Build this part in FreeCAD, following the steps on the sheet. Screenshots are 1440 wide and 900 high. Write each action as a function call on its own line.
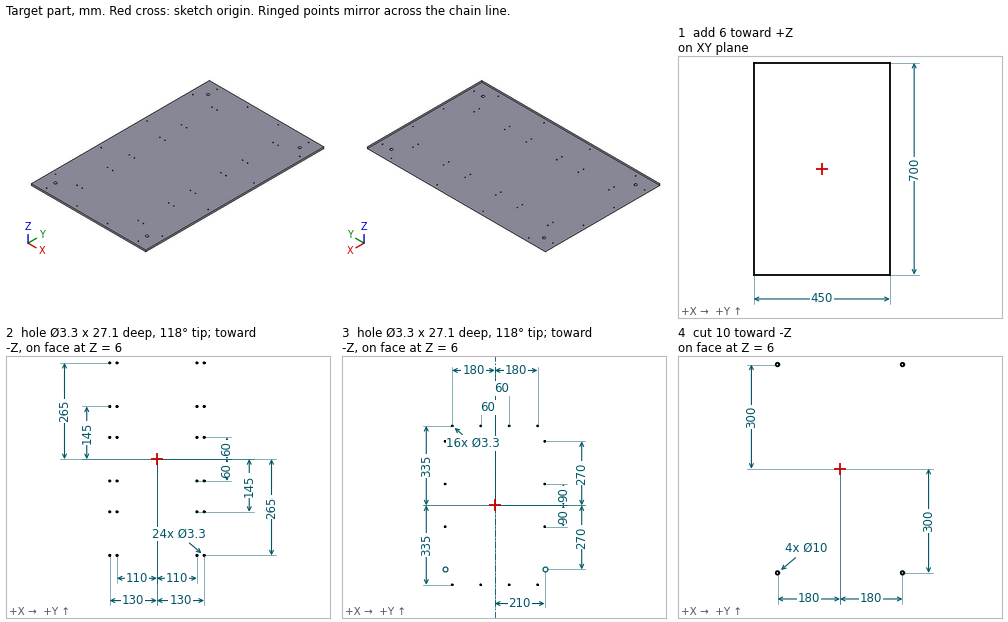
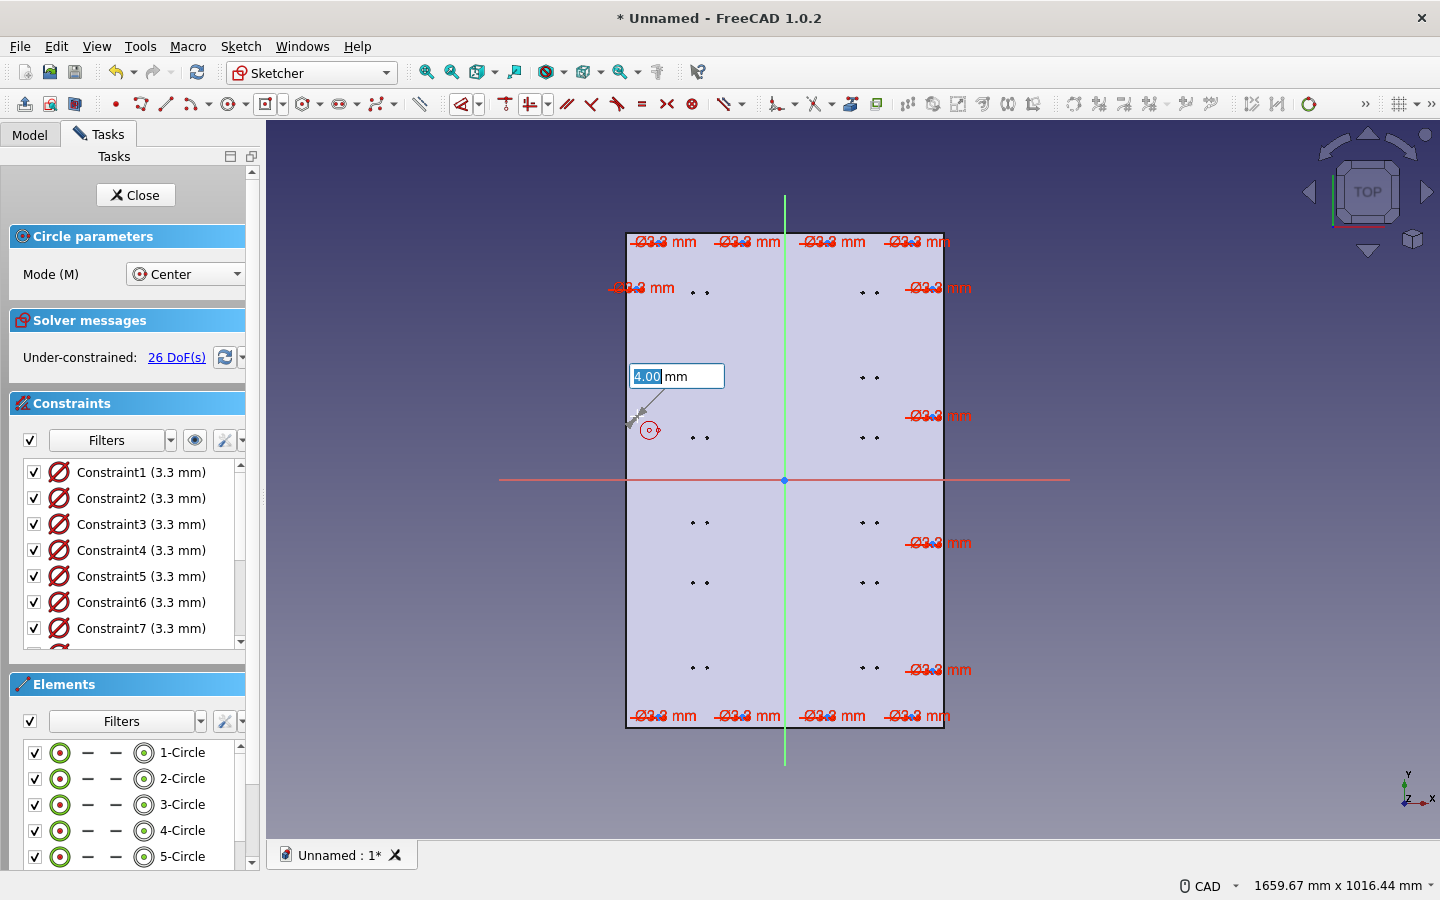
text(3.3)
key(Return)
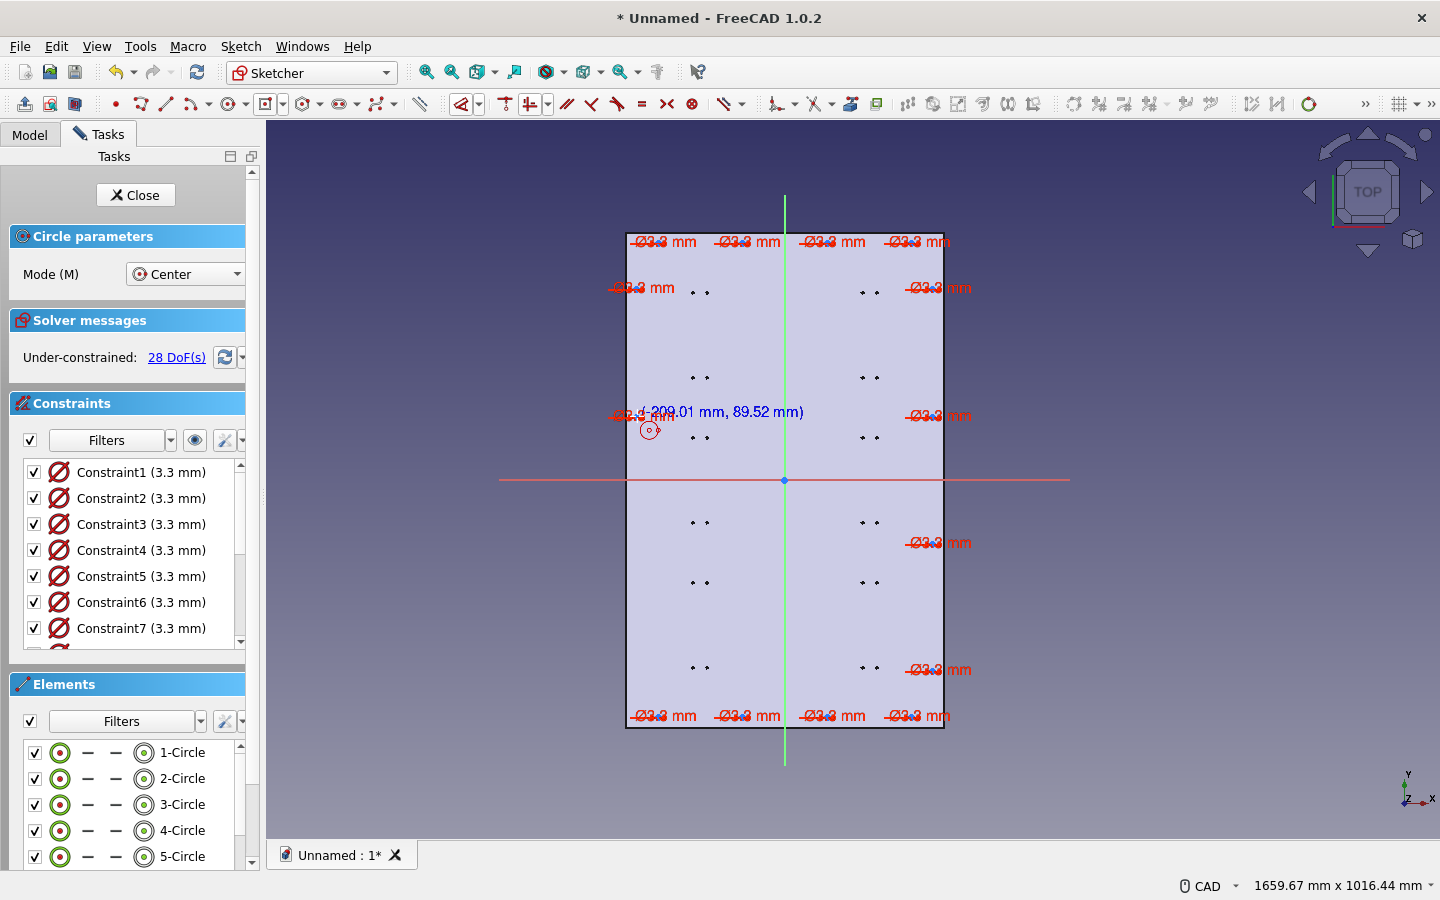
scroll(636, 544, up, 15)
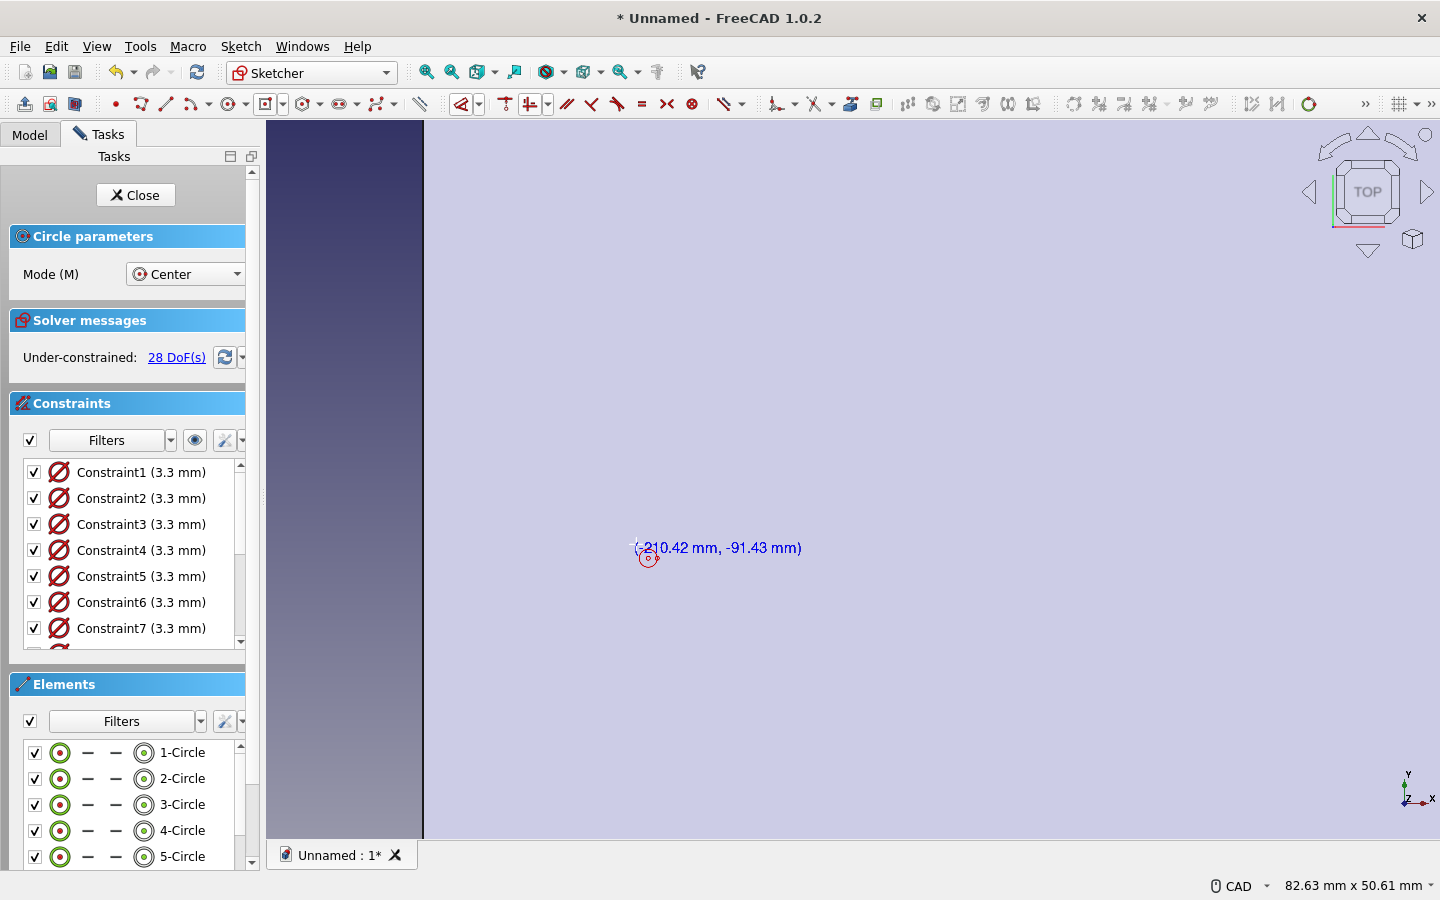
scroll(636, 544, down, 15)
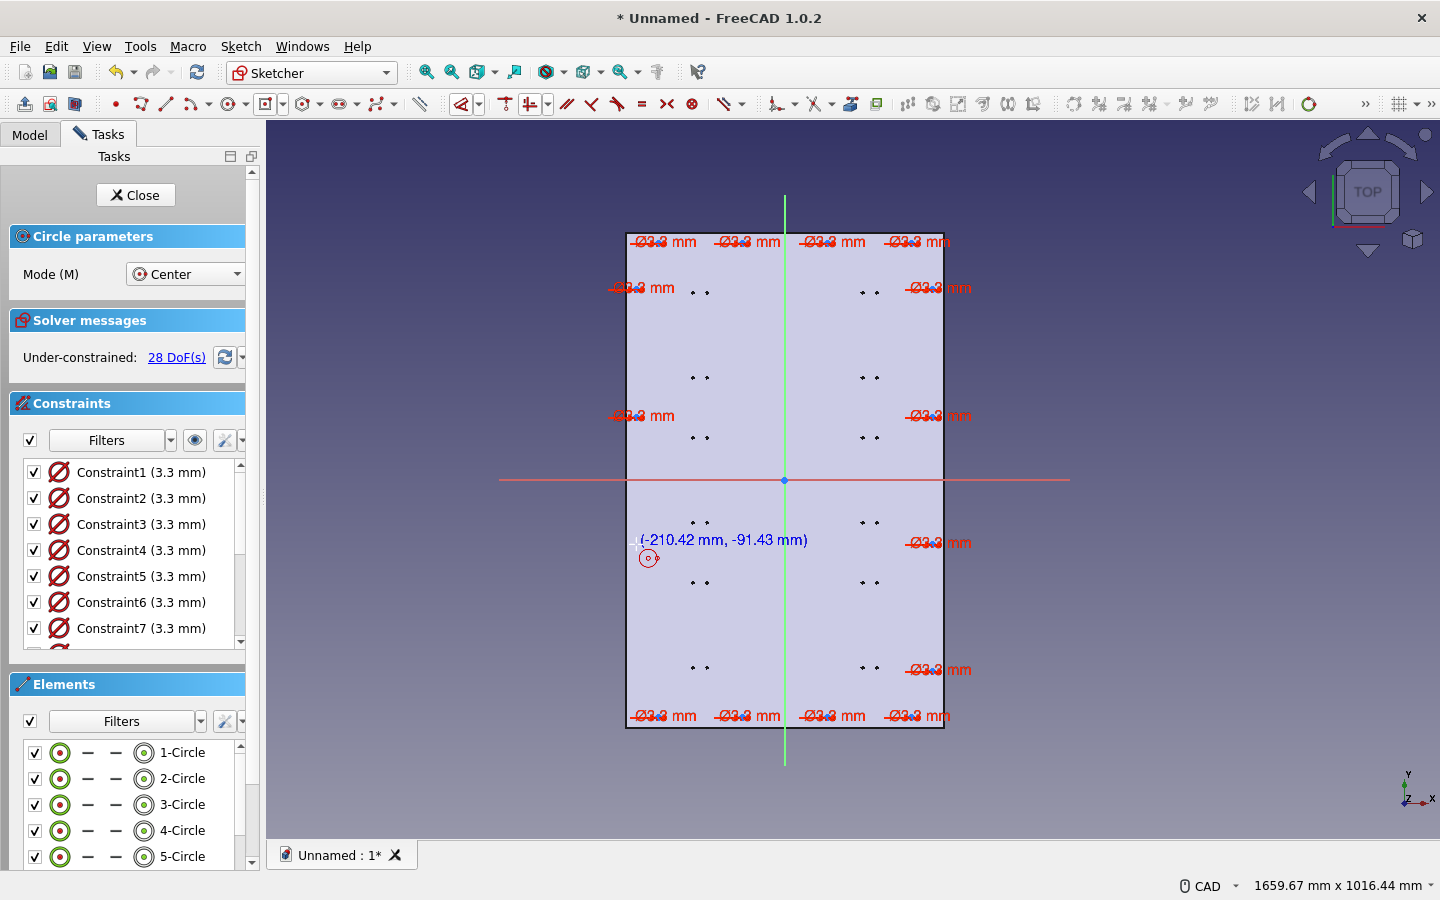
click(636, 544)
move(637, 543)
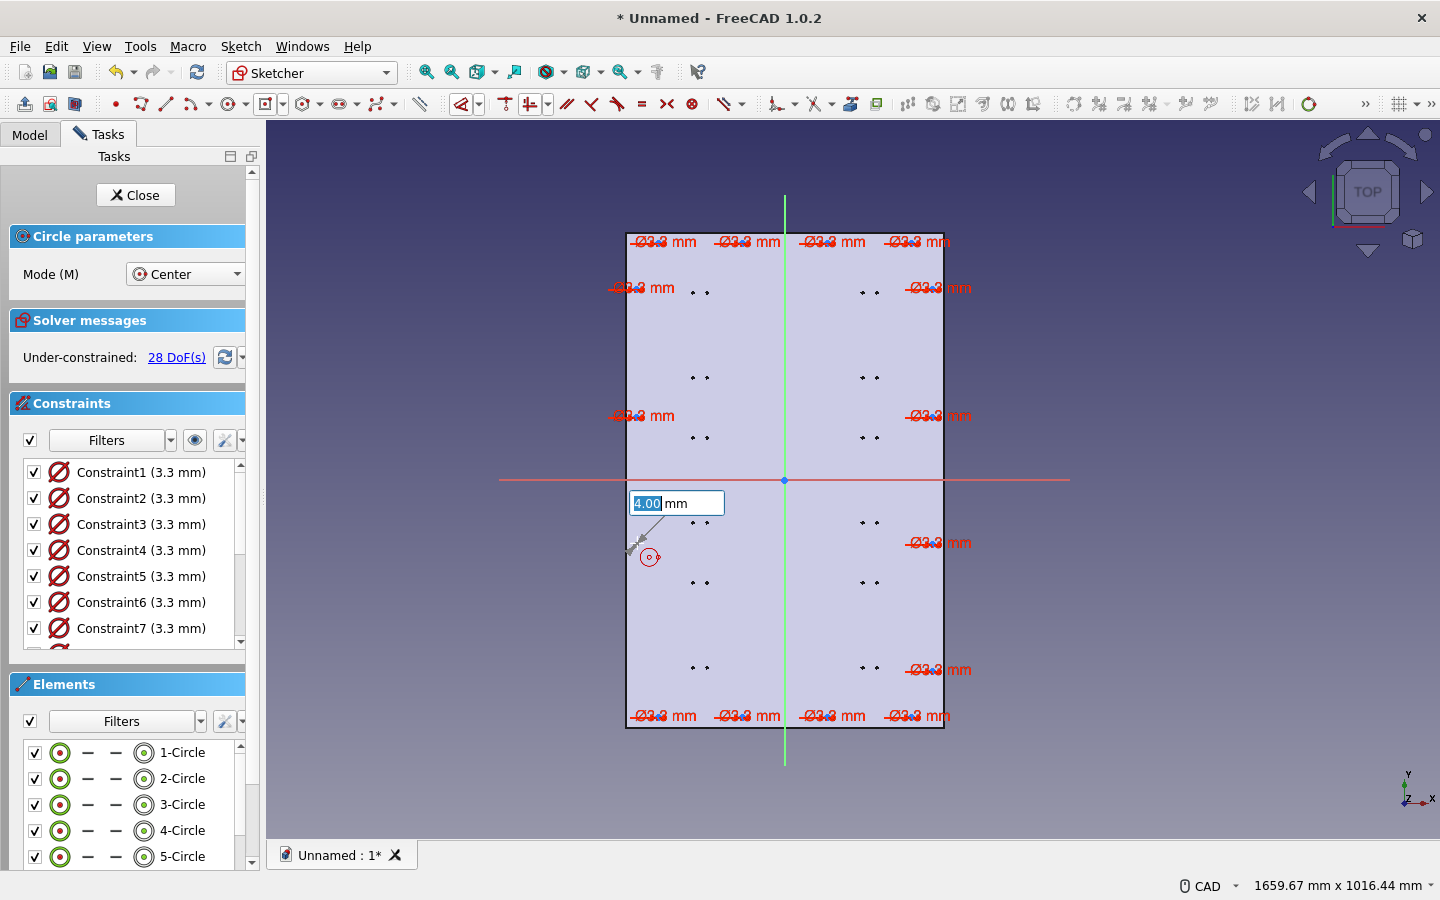
text(3.3)
key(Return)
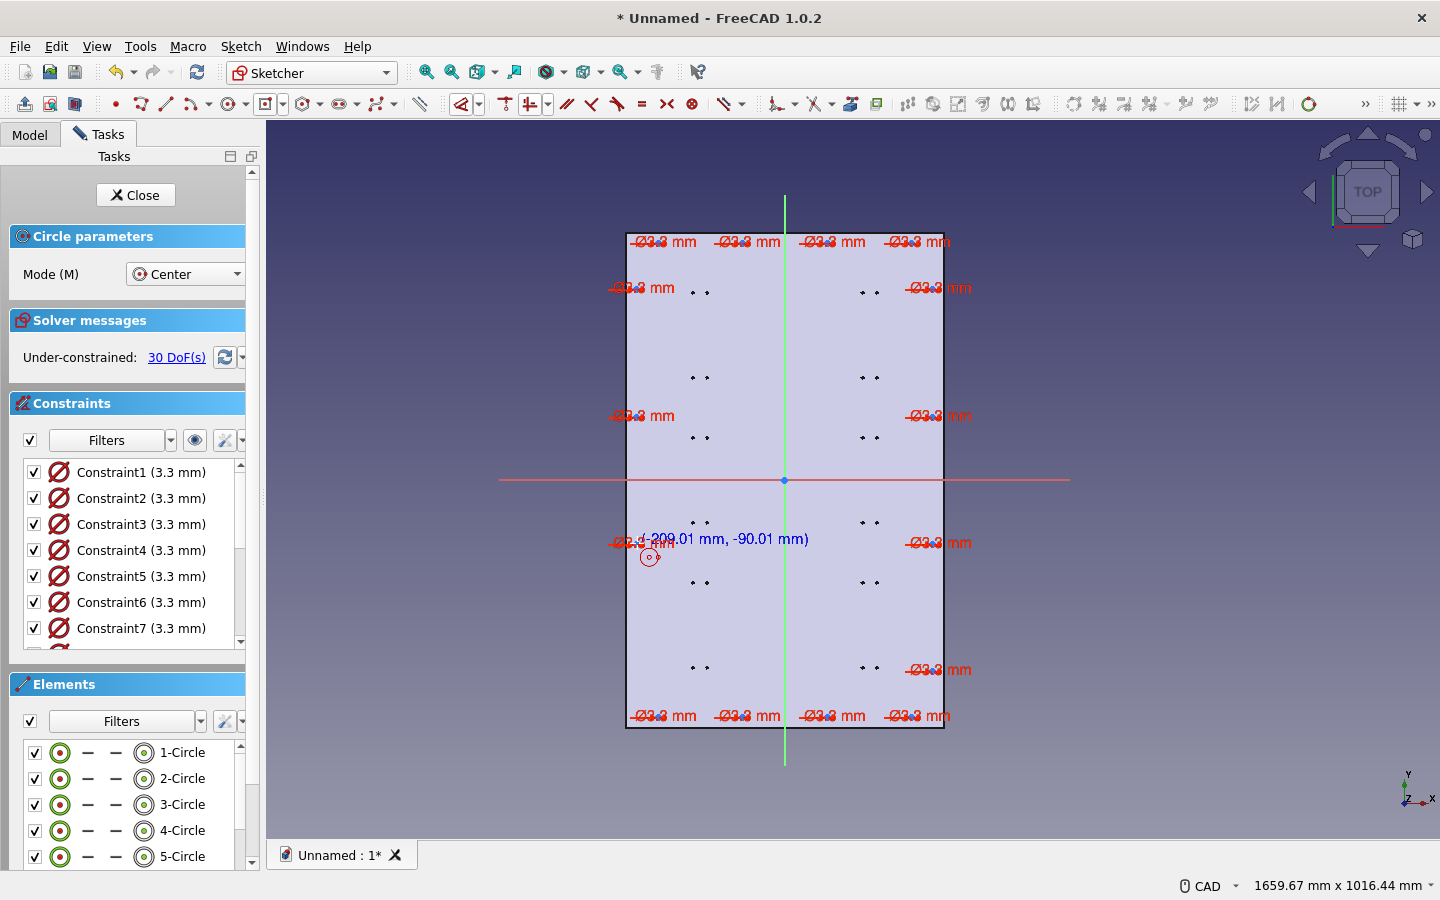
scroll(636, 671, up, 15)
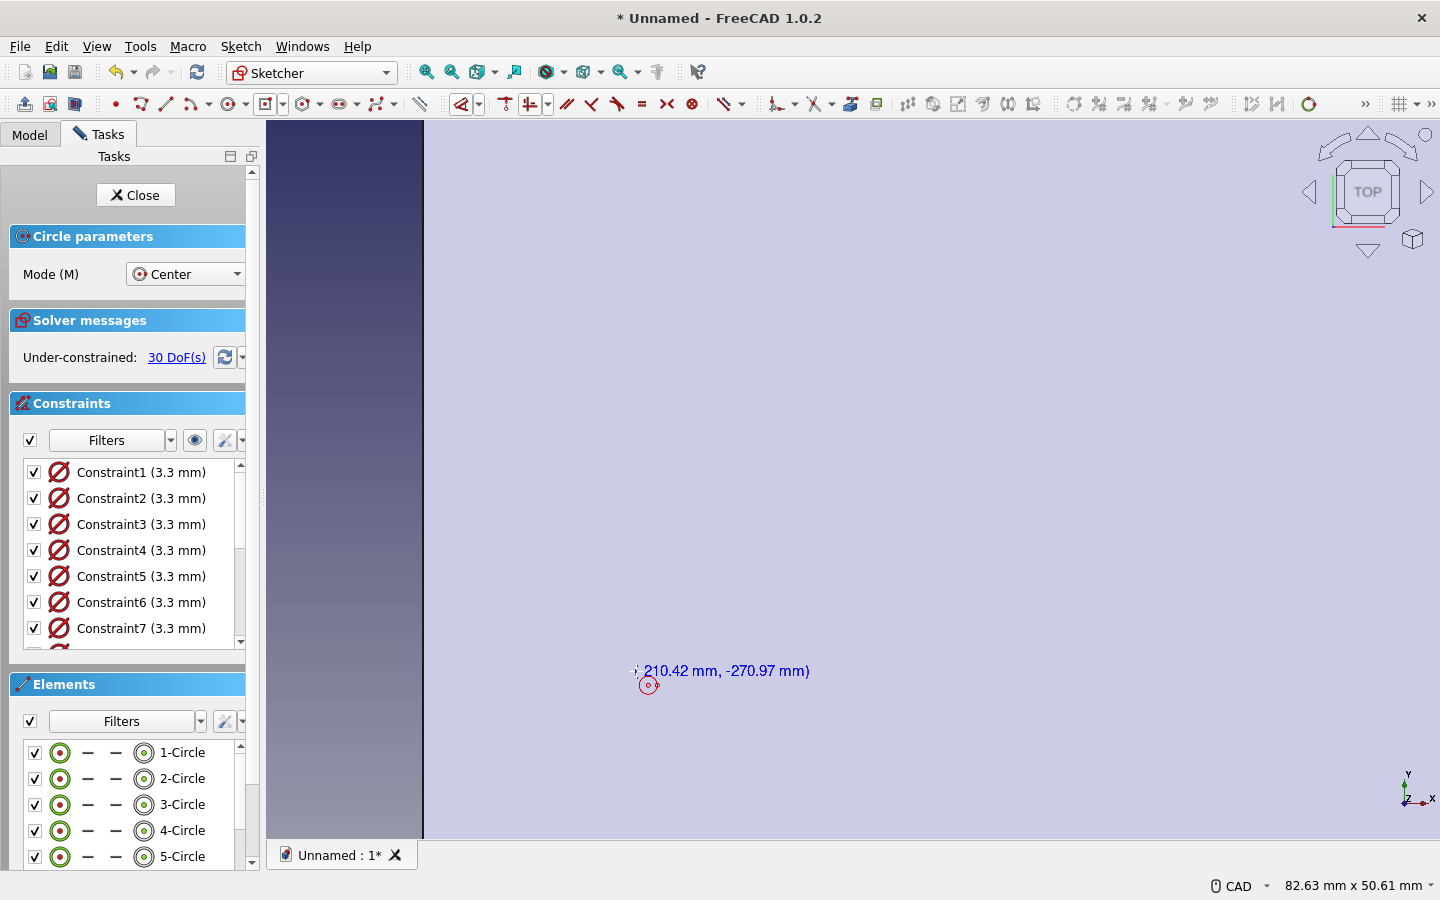
scroll(636, 671, down, 15)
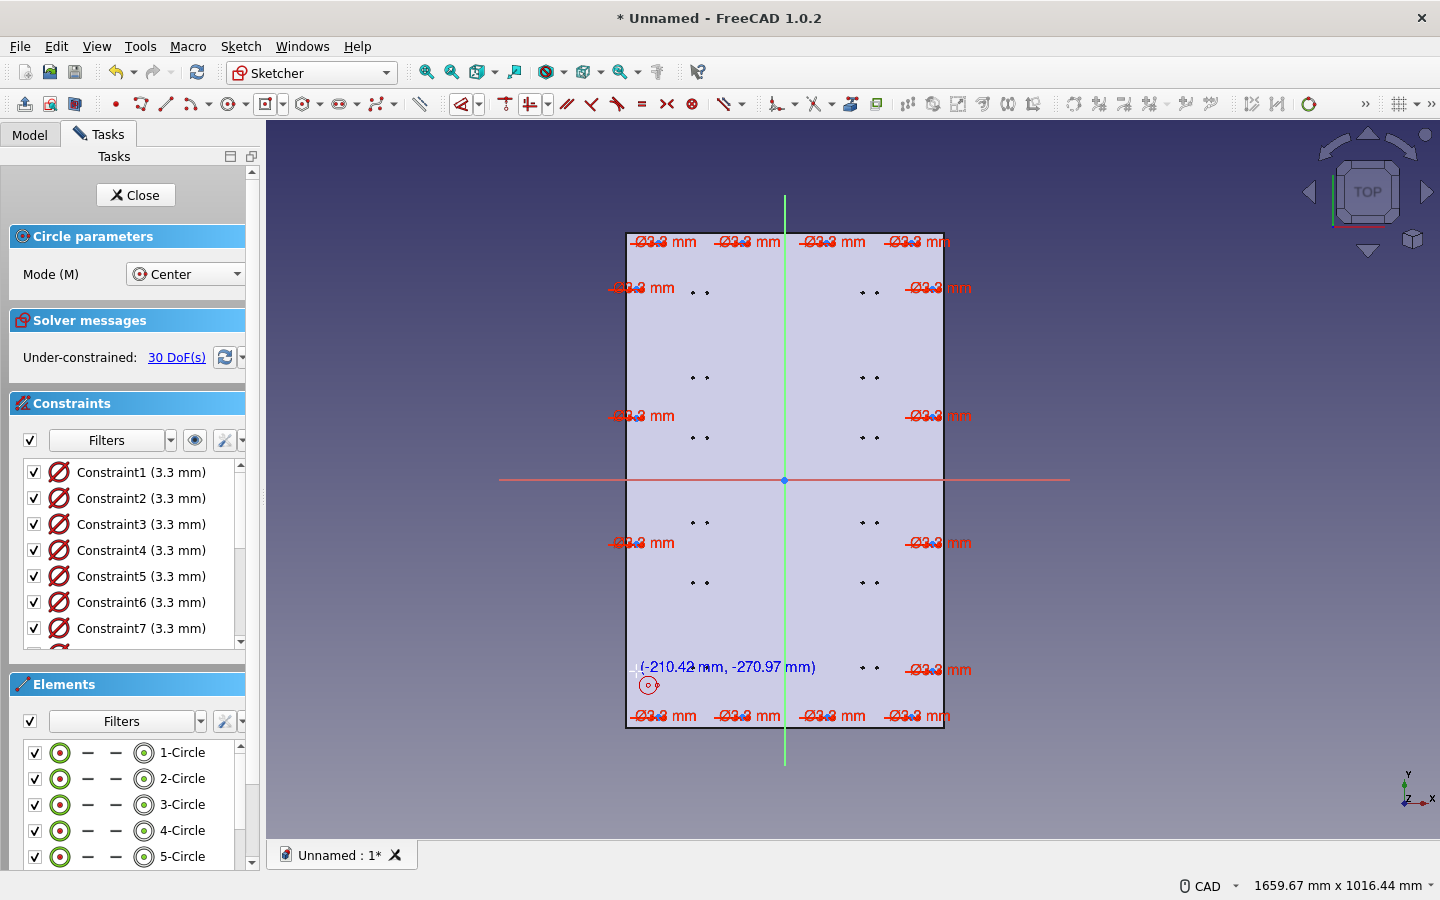
click(636, 671)
move(637, 670)